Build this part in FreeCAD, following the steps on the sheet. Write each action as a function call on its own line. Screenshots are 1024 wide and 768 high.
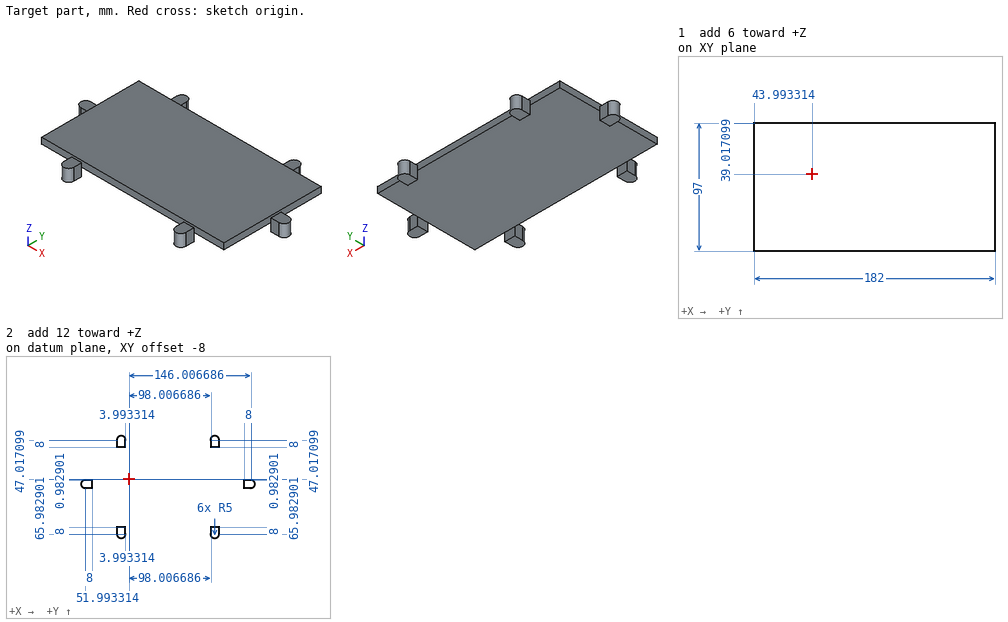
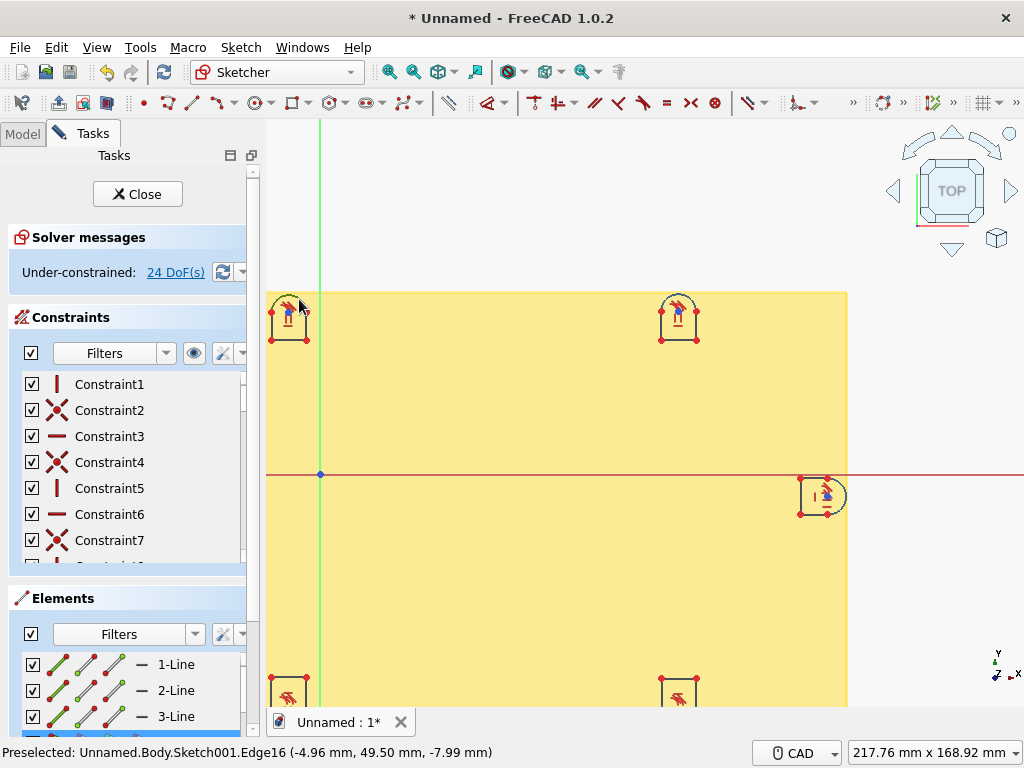
scroll(689, 298, down, 3)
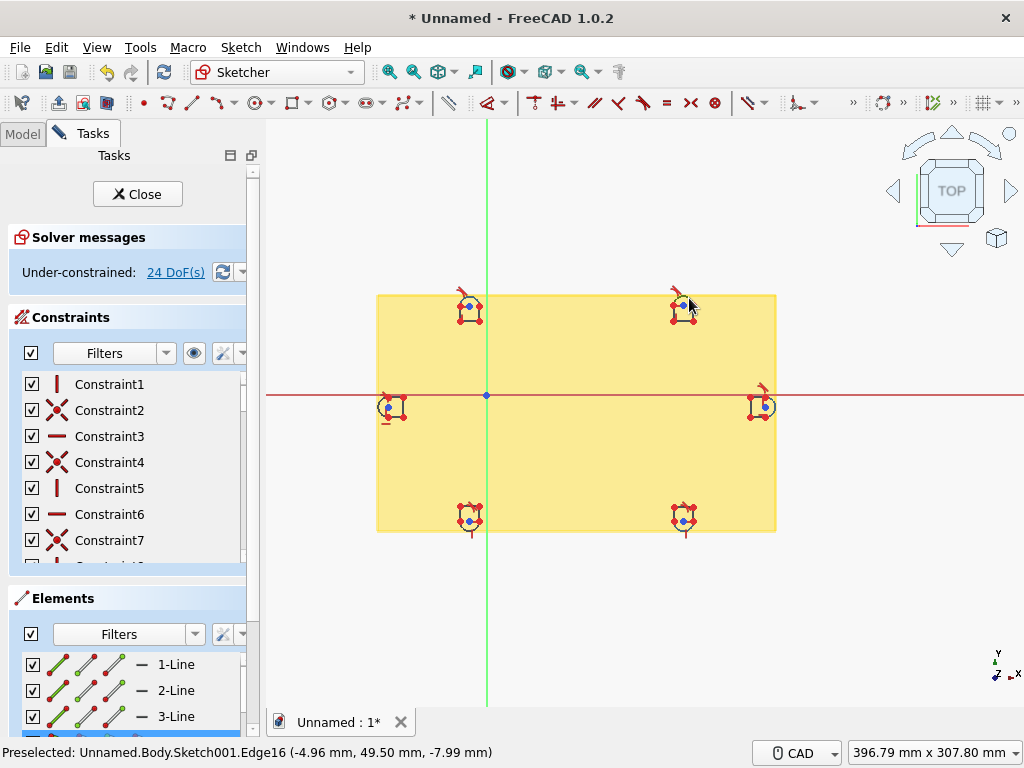
scroll(380, 401, up, 5)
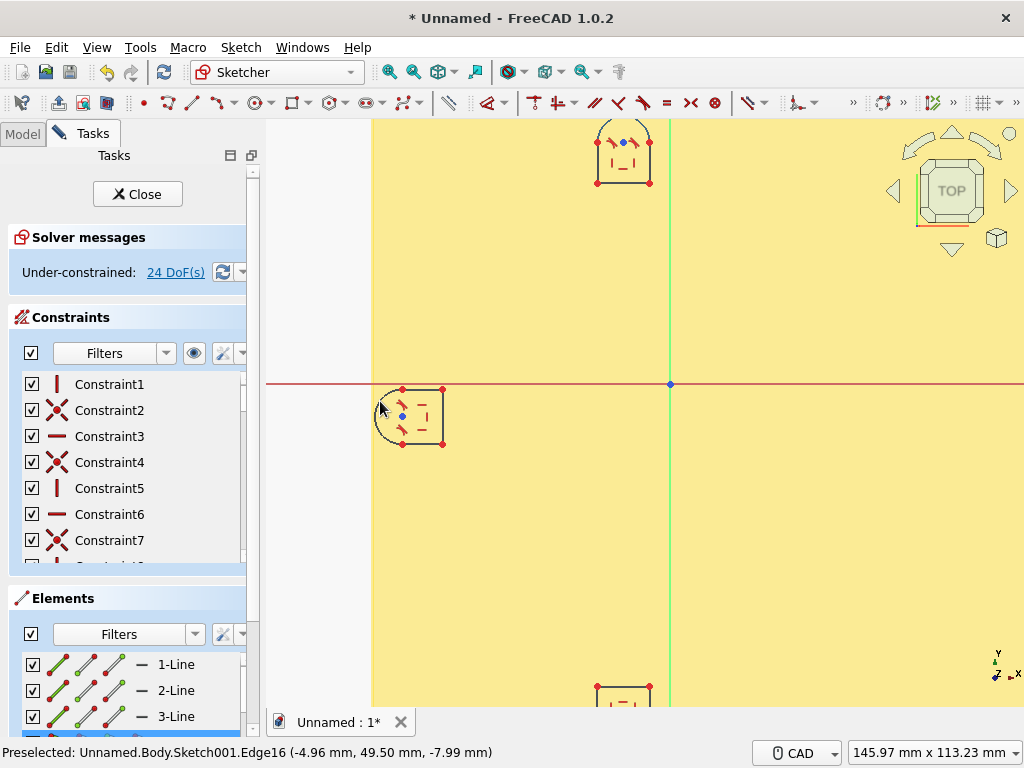
click(380, 401)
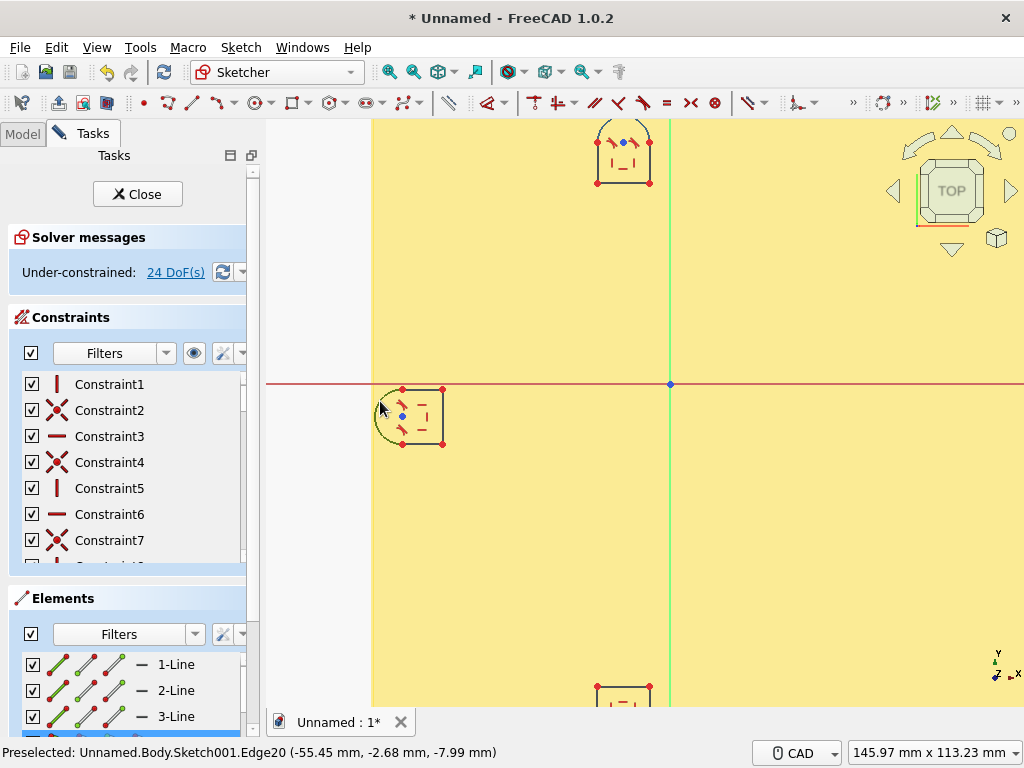
scroll(380, 401, down, 5)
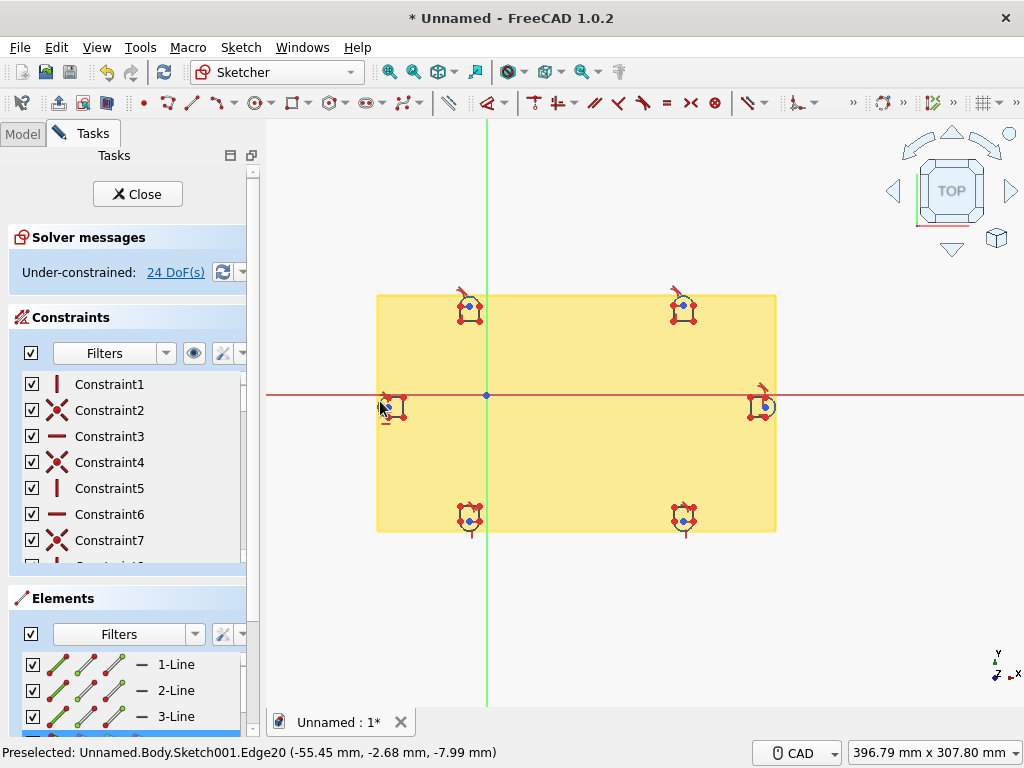
scroll(464, 529, up, 3)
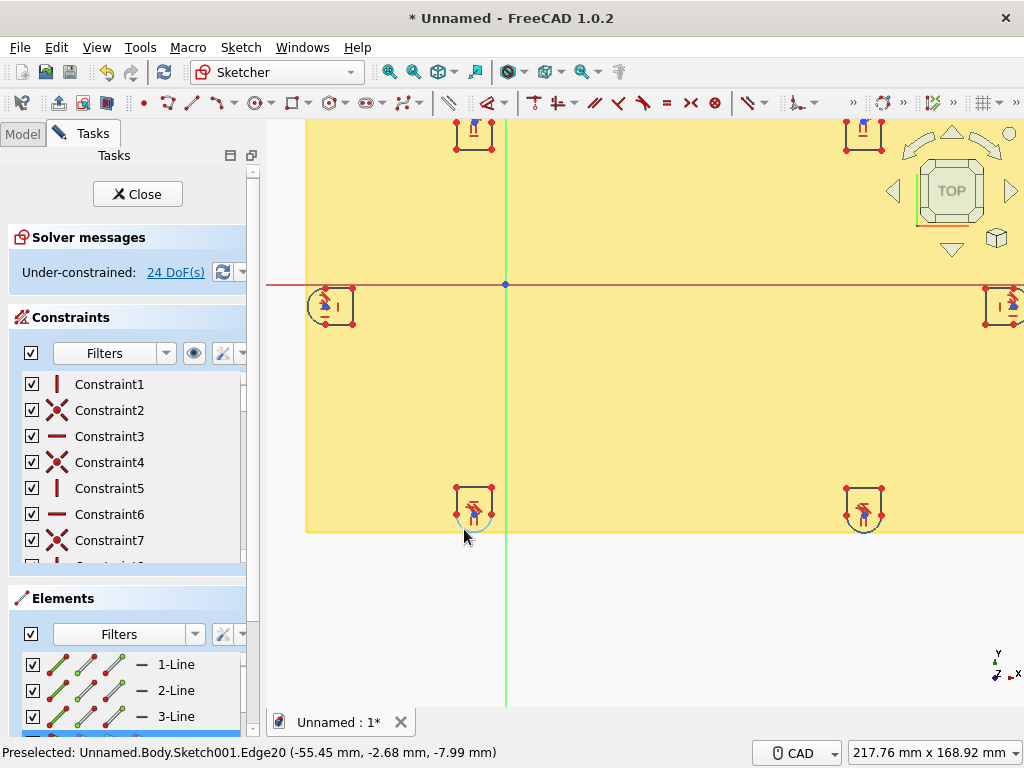
click(464, 529)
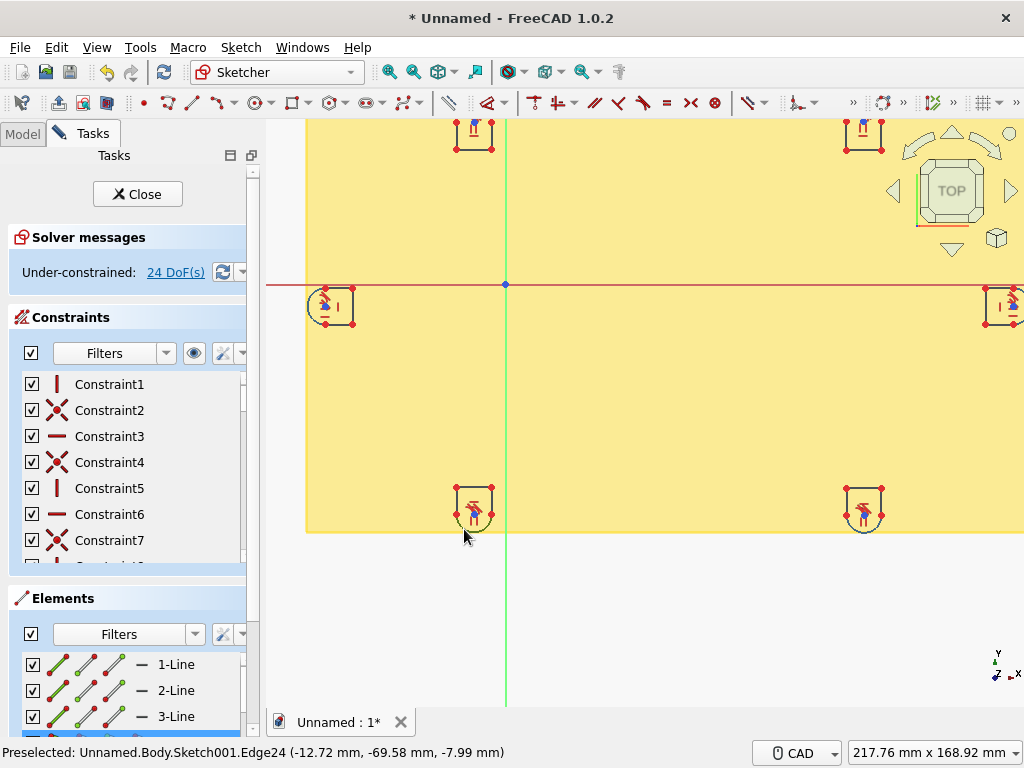
click(668, 104)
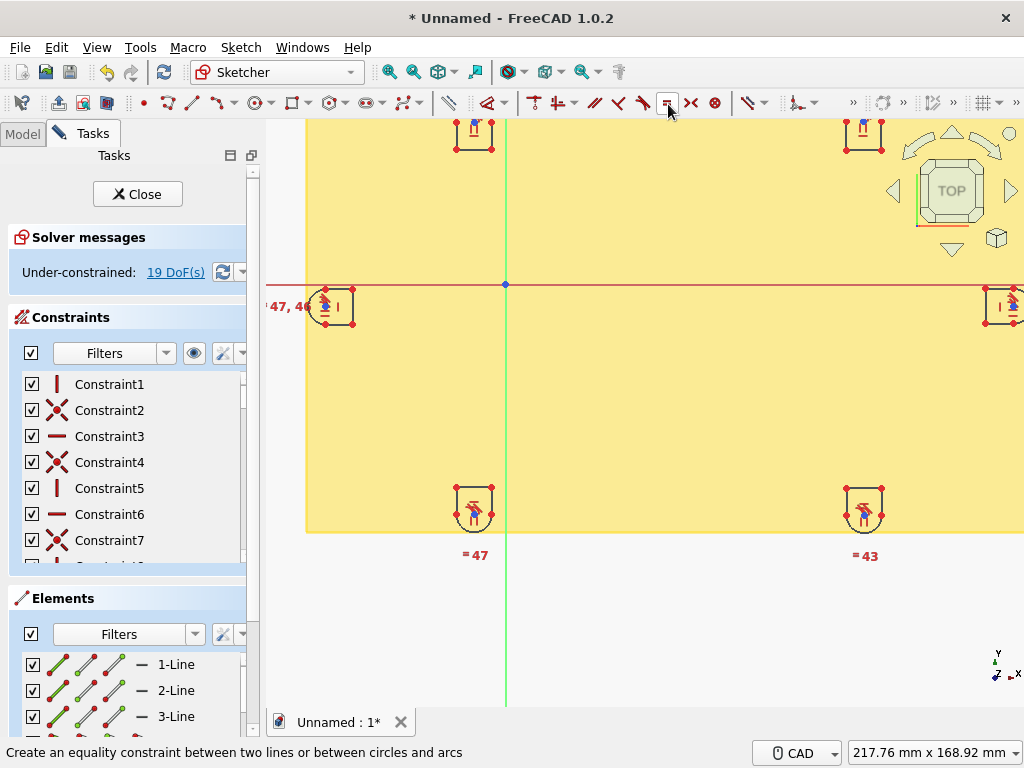
click(488, 104)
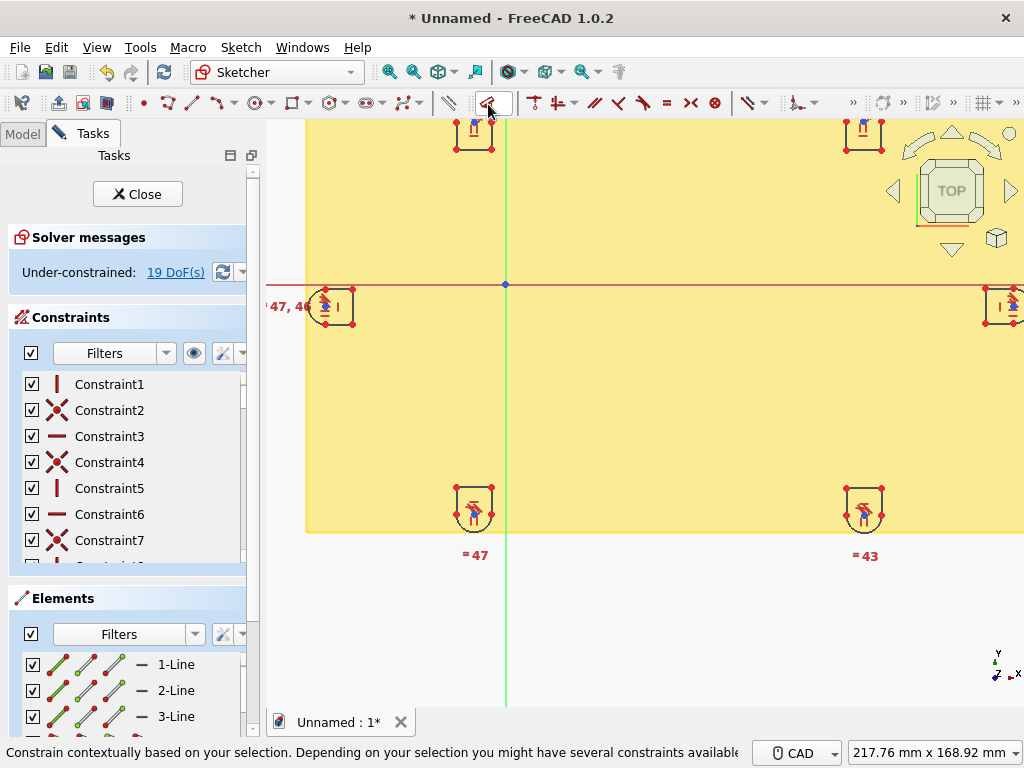
scroll(854, 530, up, 5)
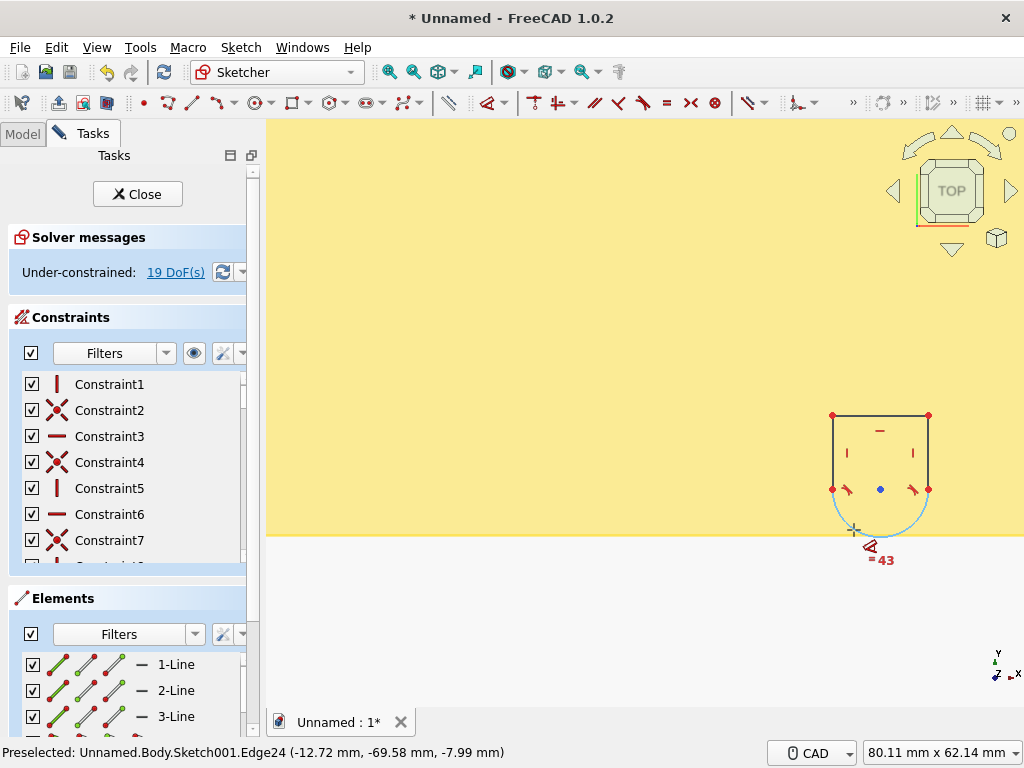
click(852, 528)
click(833, 554)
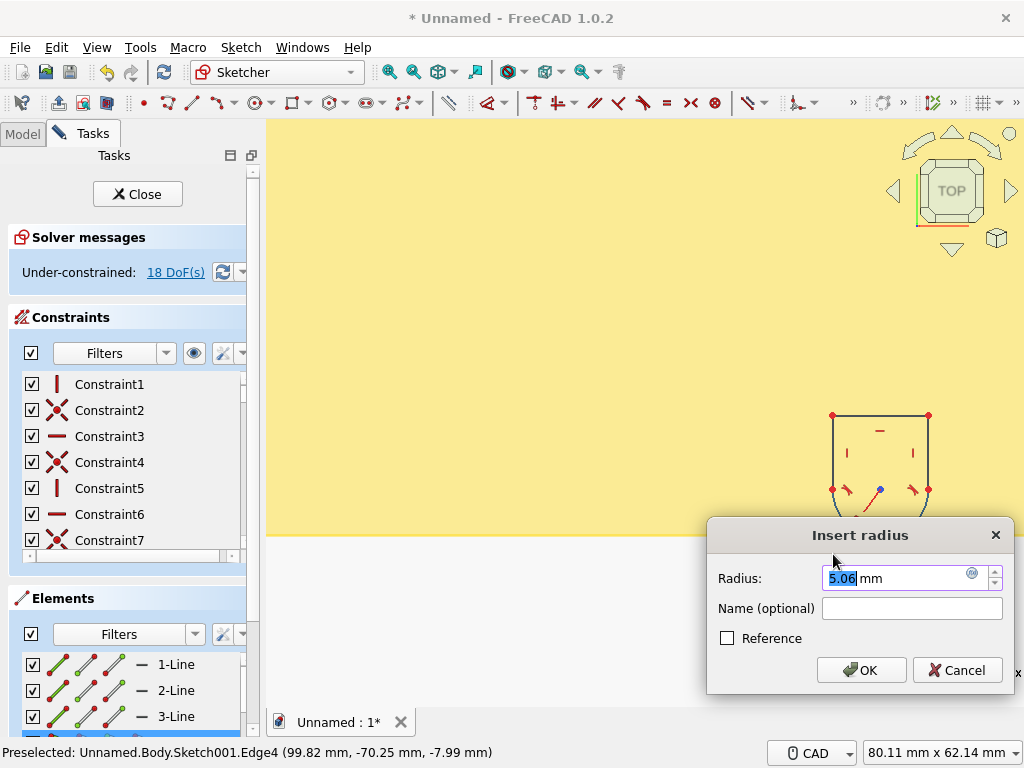
text(5)
key(Return)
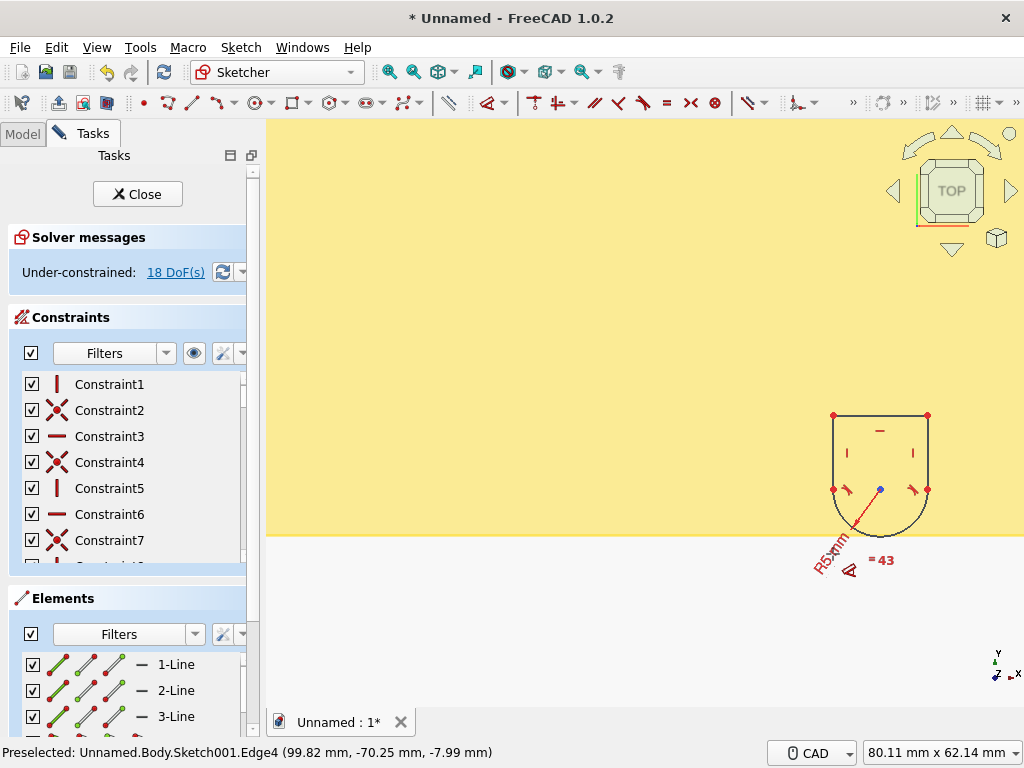
scroll(634, 530, down, 8)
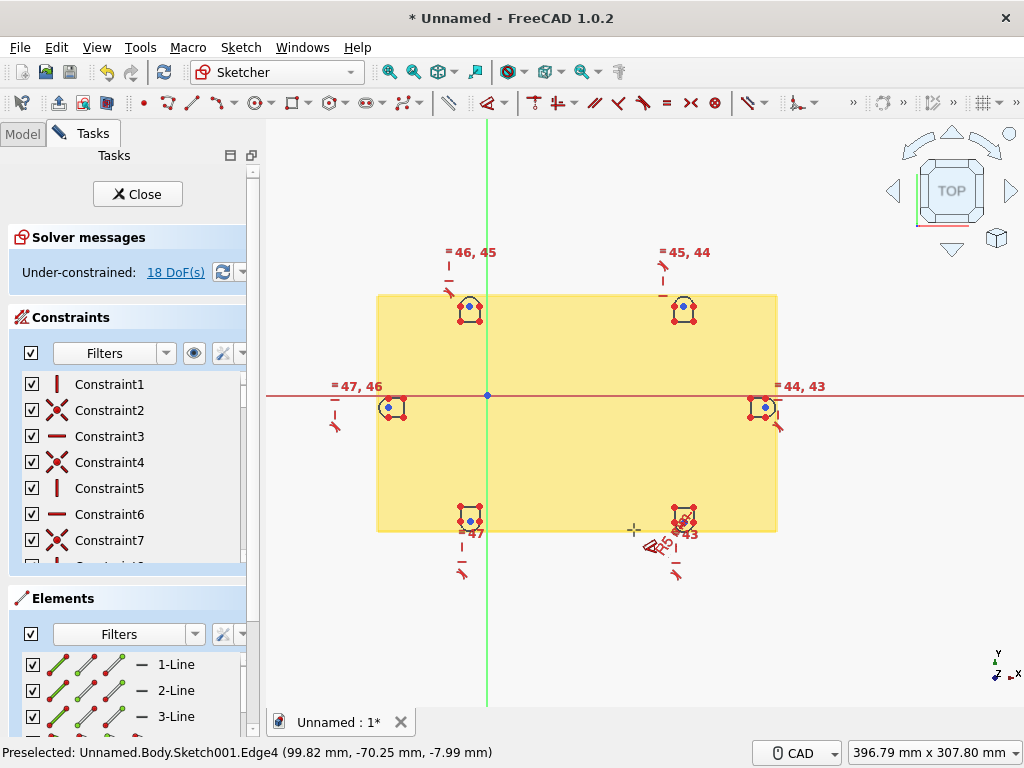
scroll(694, 518, up, 6)